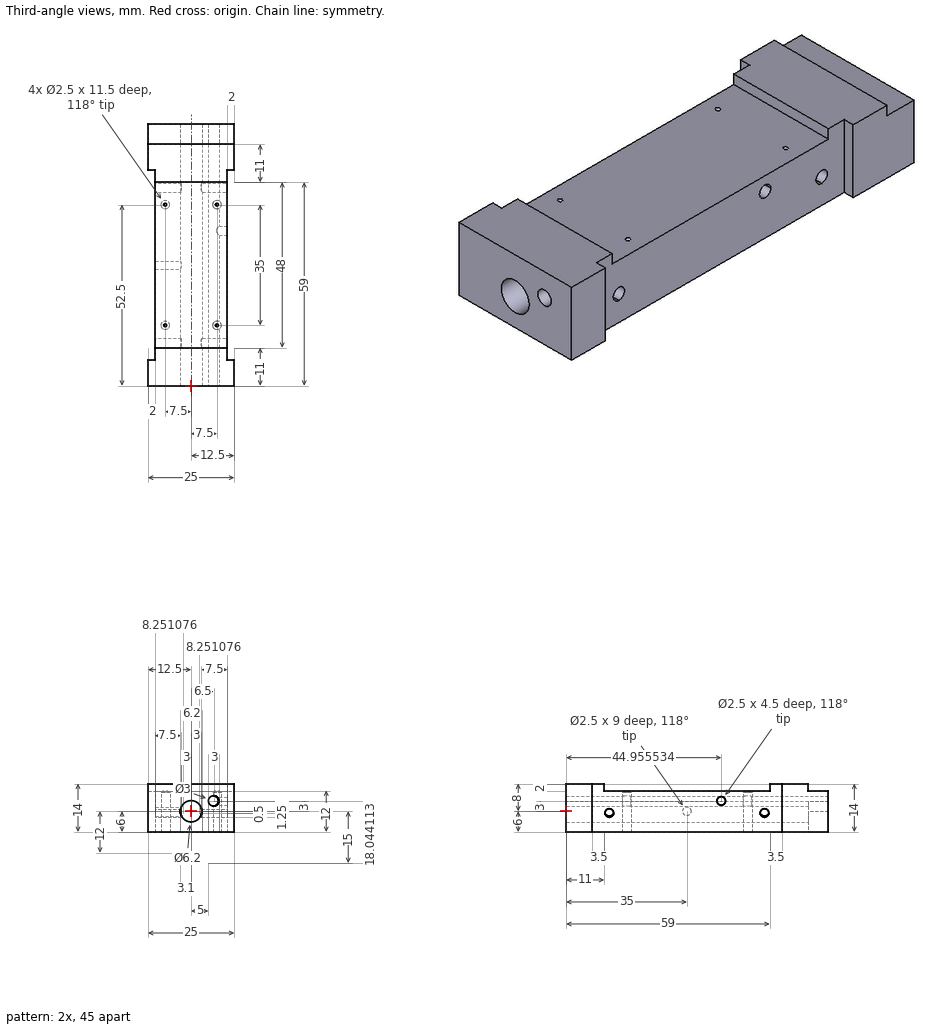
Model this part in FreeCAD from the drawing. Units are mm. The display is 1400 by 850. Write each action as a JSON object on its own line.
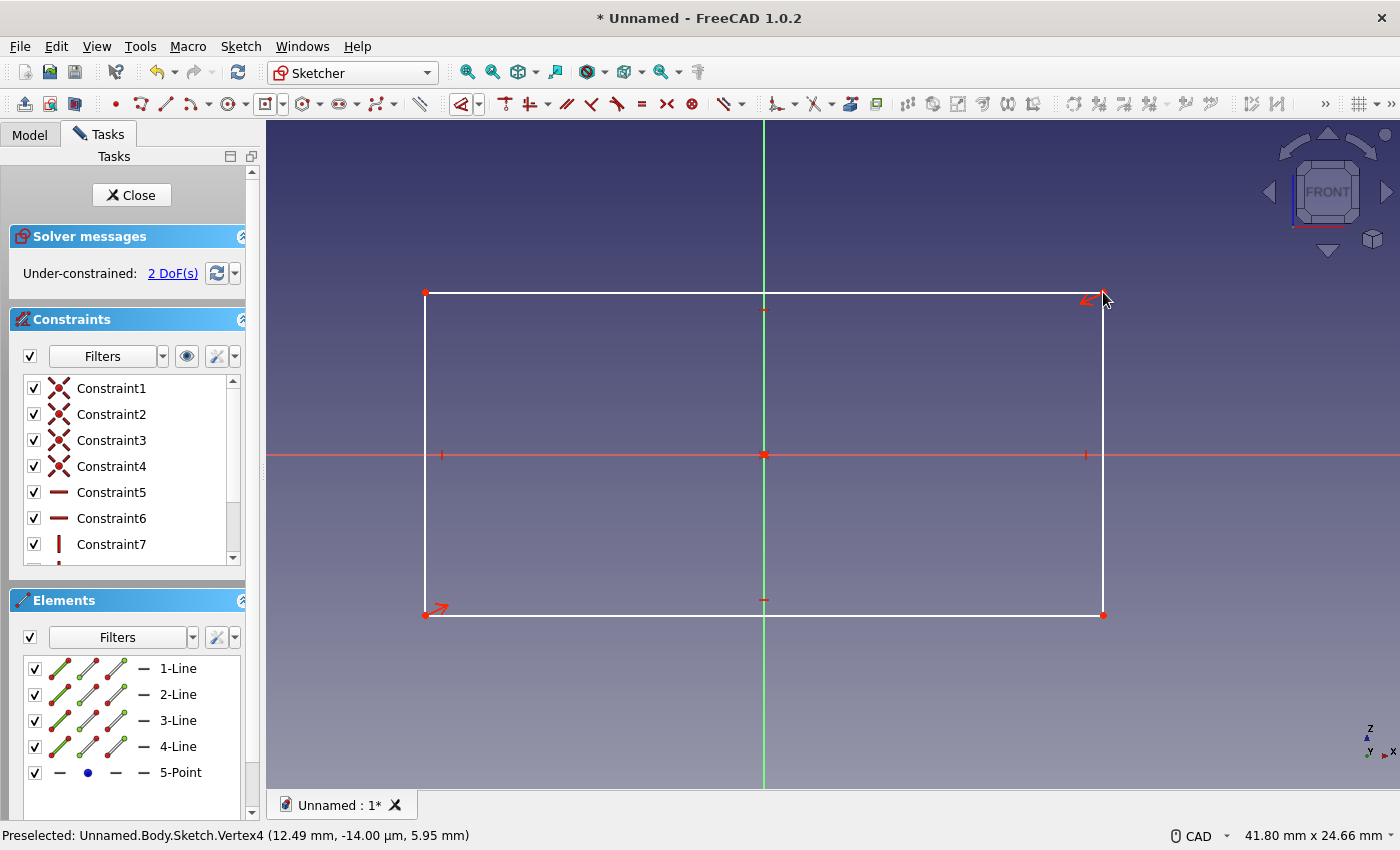
{"action": "left_click", "coordinate": [460, 104]}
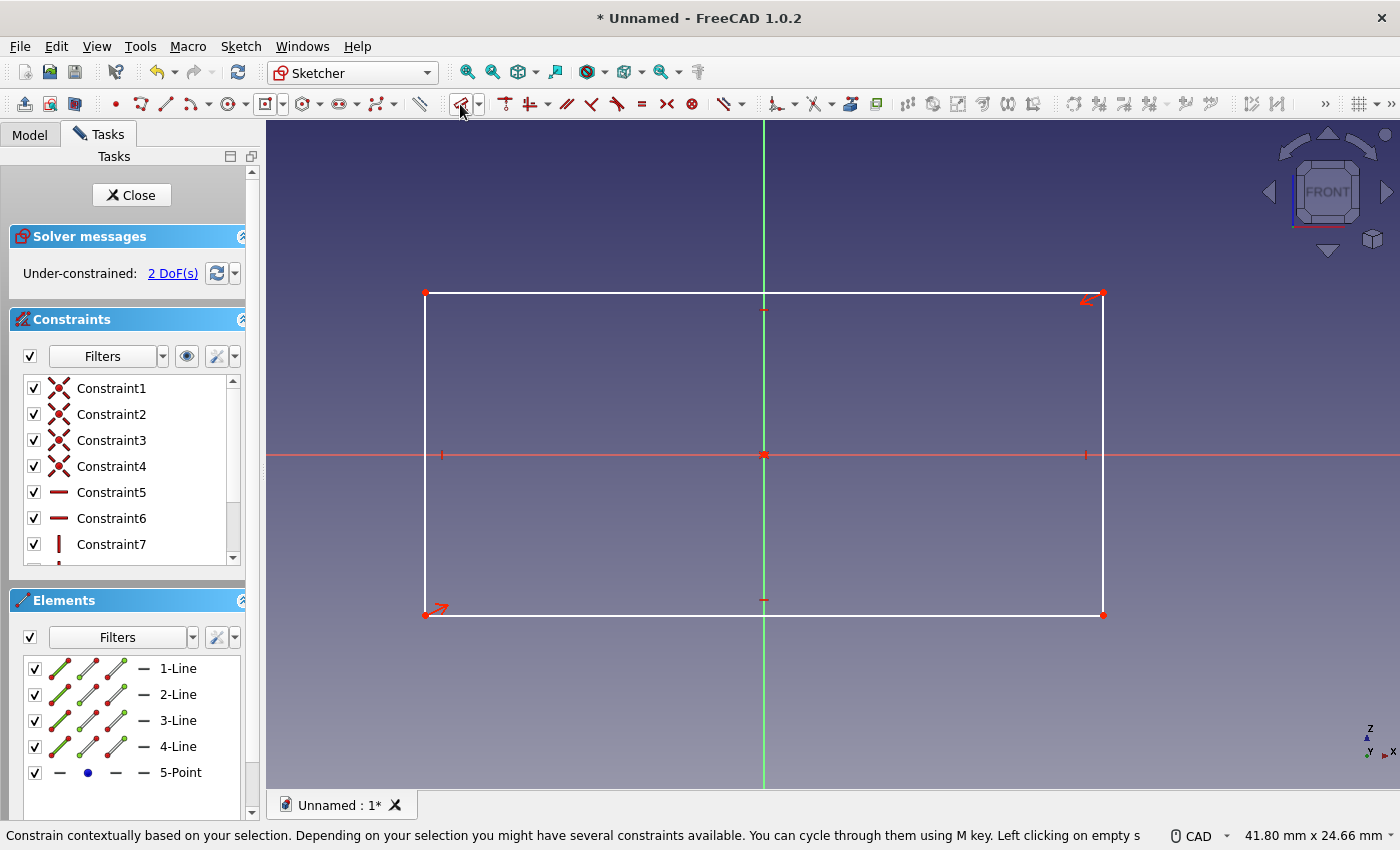
{"action": "left_click", "coordinate": [629, 616]}
{"action": "left_click", "coordinate": [608, 650]}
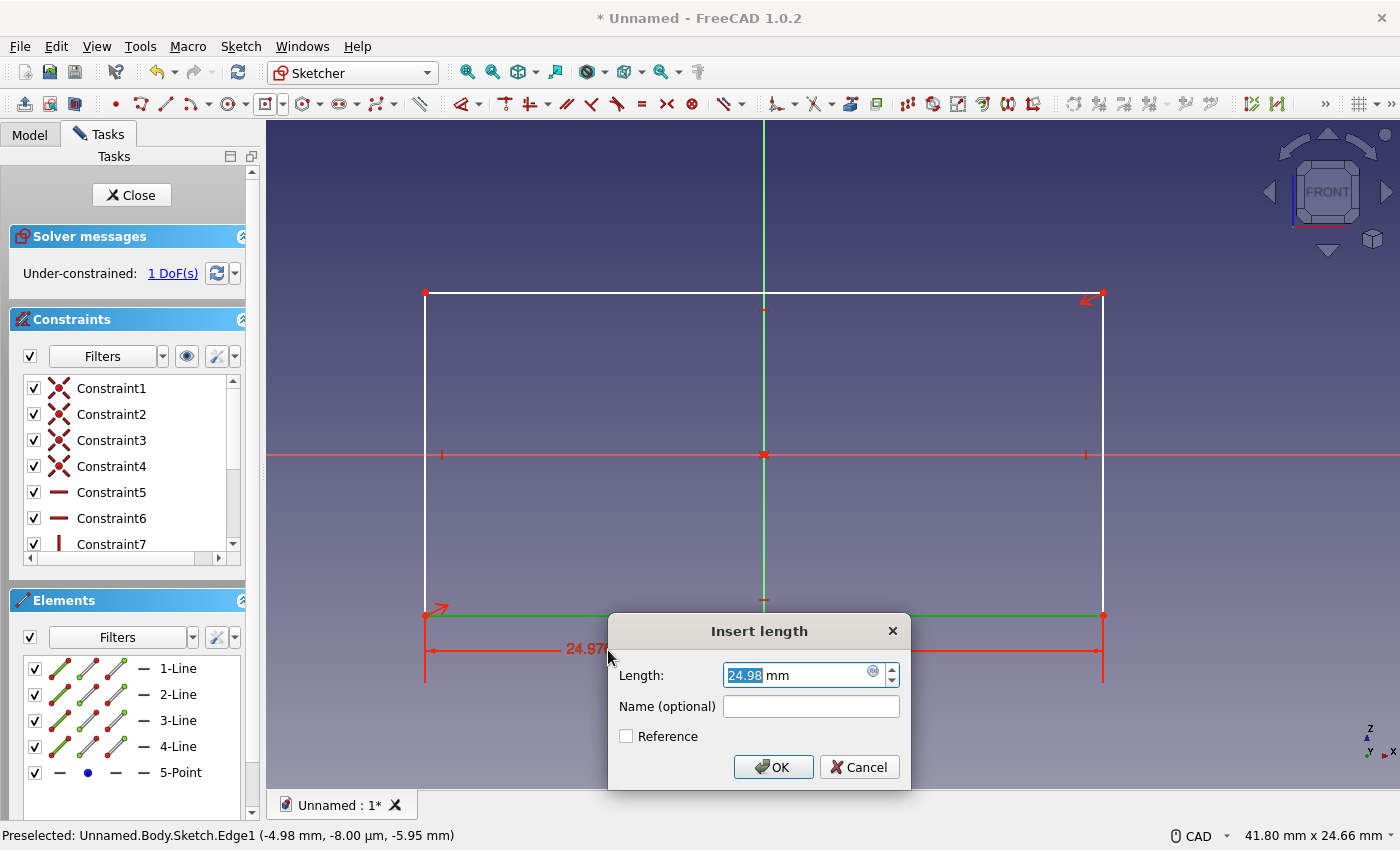
{"action": "type", "text": "25"}
{"action": "key", "text": "Return"}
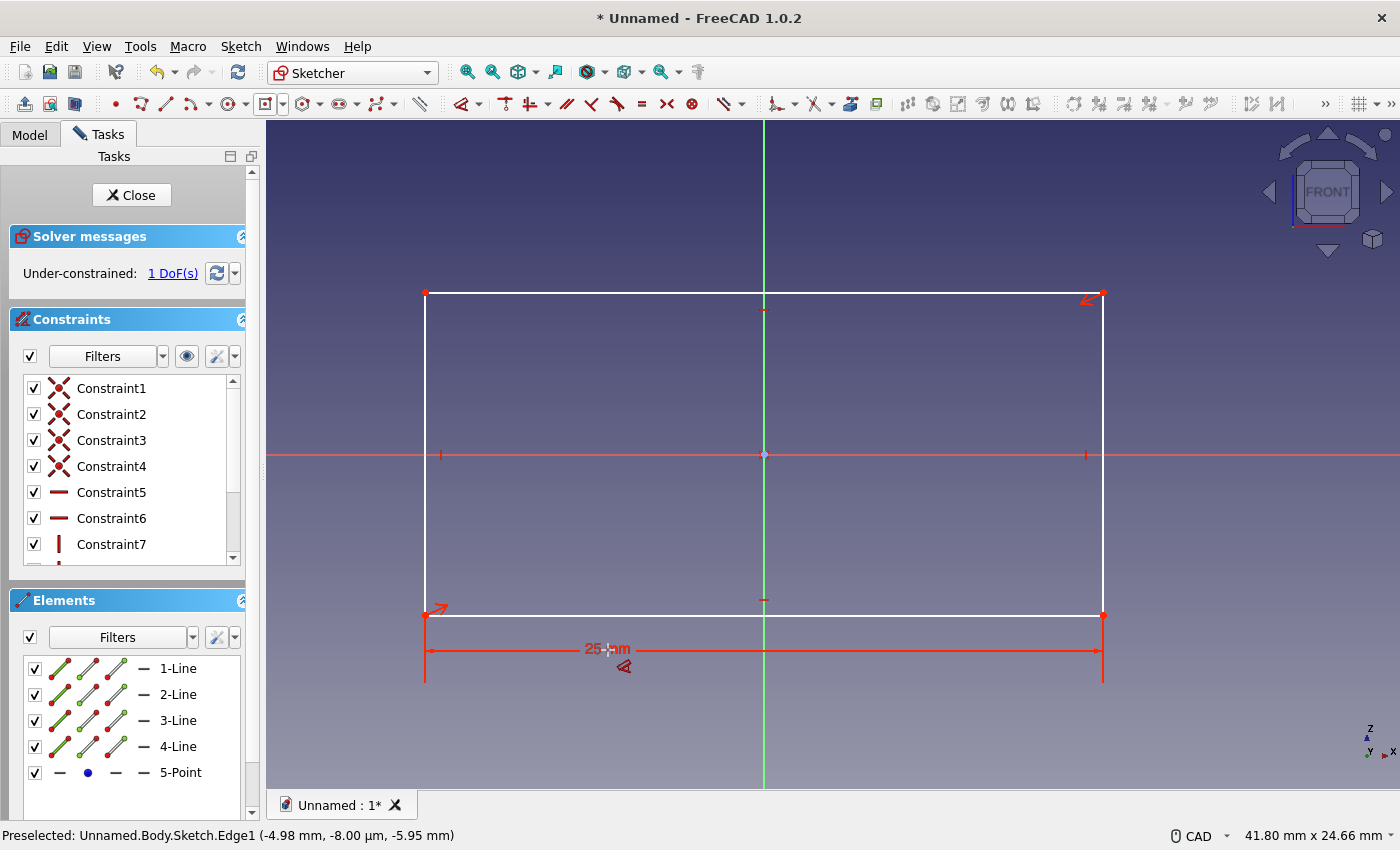
{"action": "left_click", "coordinate": [1103, 519]}
{"action": "left_click", "coordinate": [1137, 380]}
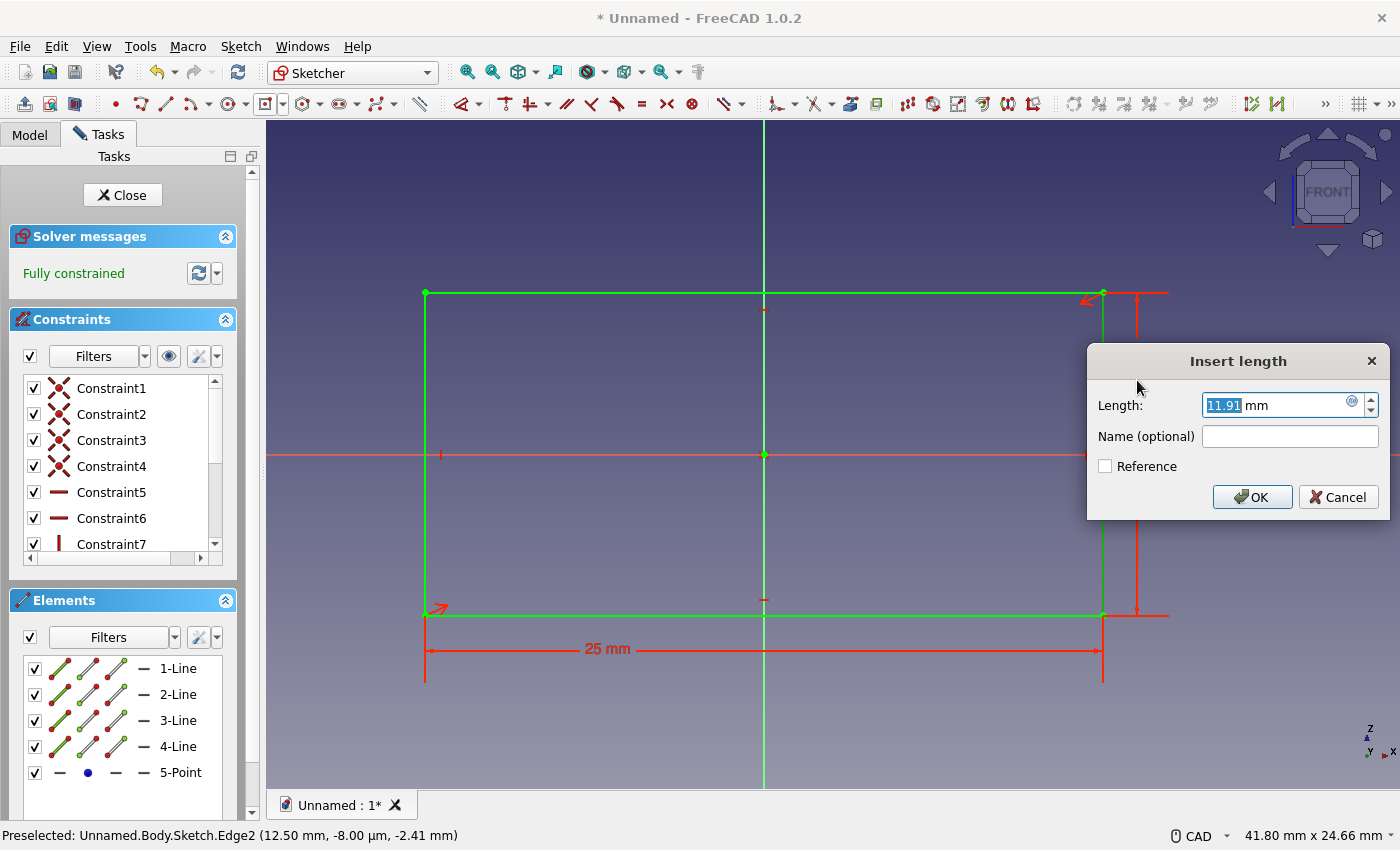
{"action": "type", "text": "12"}
{"action": "key", "text": "Return"}
{"action": "key", "text": "Escape"}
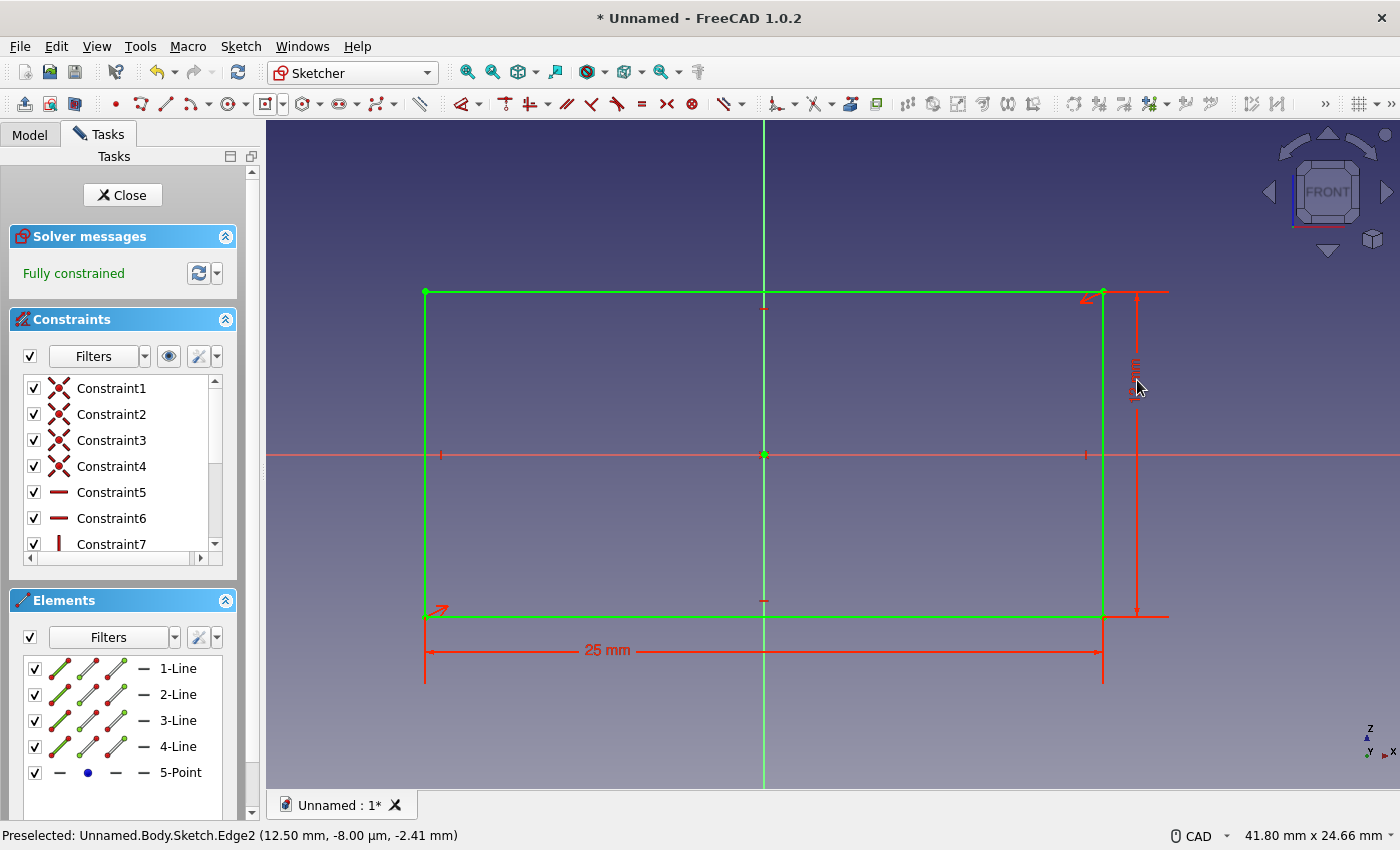
{"action": "left_click", "coordinate": [123, 195]}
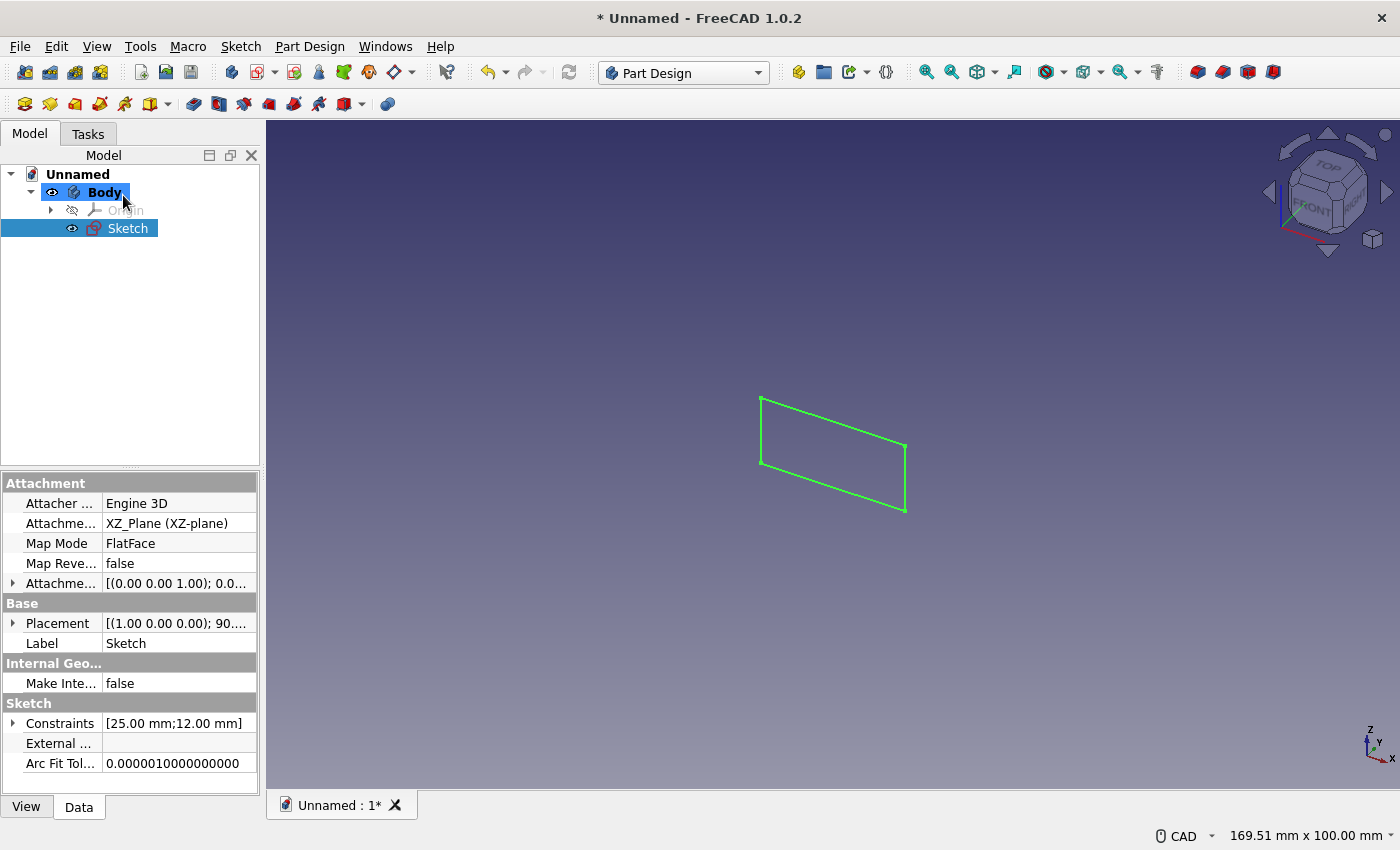
{"action": "left_click", "coordinate": [25, 104]}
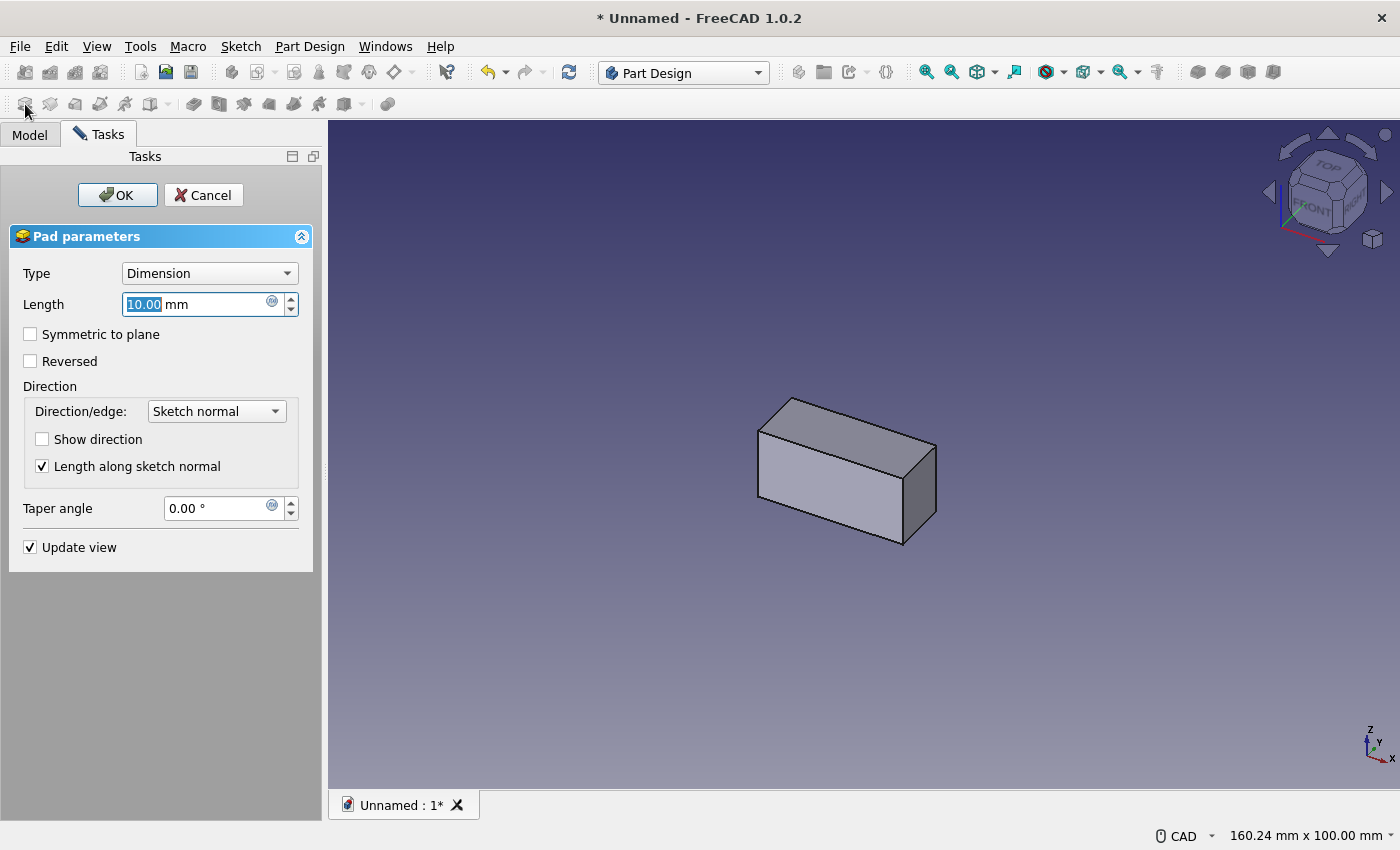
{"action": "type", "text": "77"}
{"action": "key", "text": "Tab"}